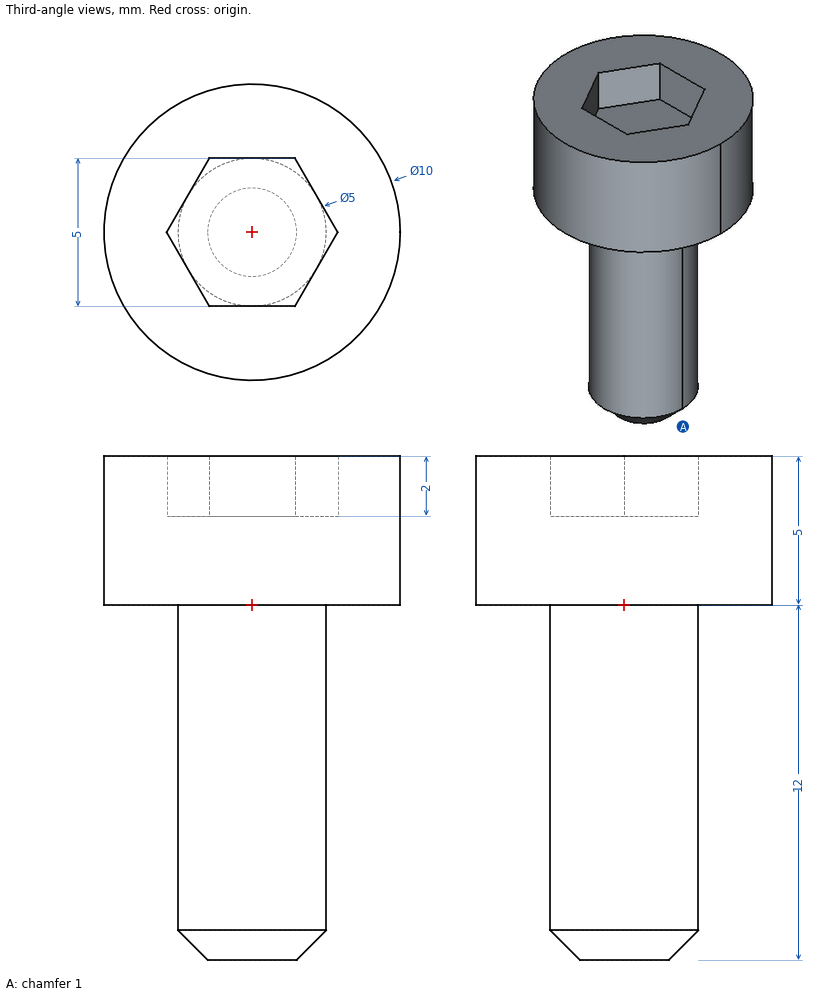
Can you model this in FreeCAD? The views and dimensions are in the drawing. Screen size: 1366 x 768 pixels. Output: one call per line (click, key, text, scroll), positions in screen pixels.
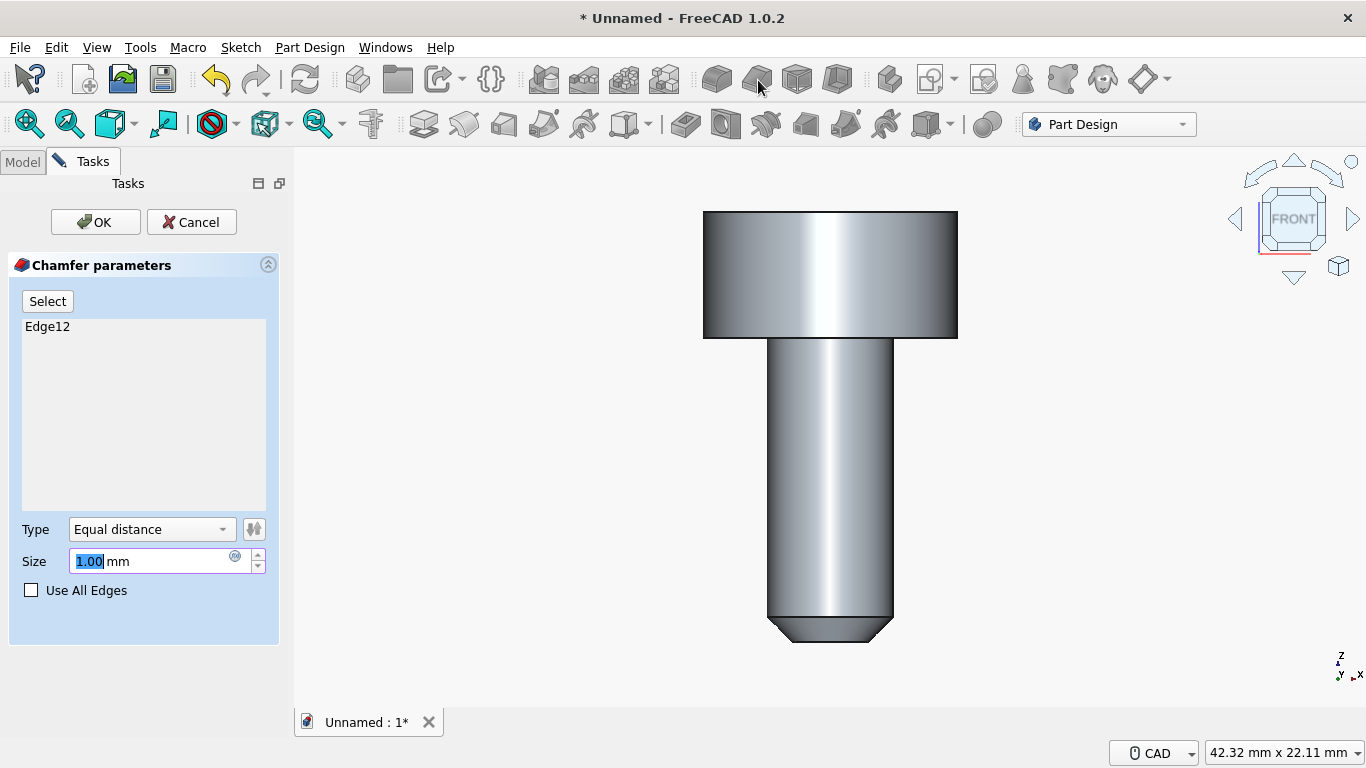
text(1)
key(Tab)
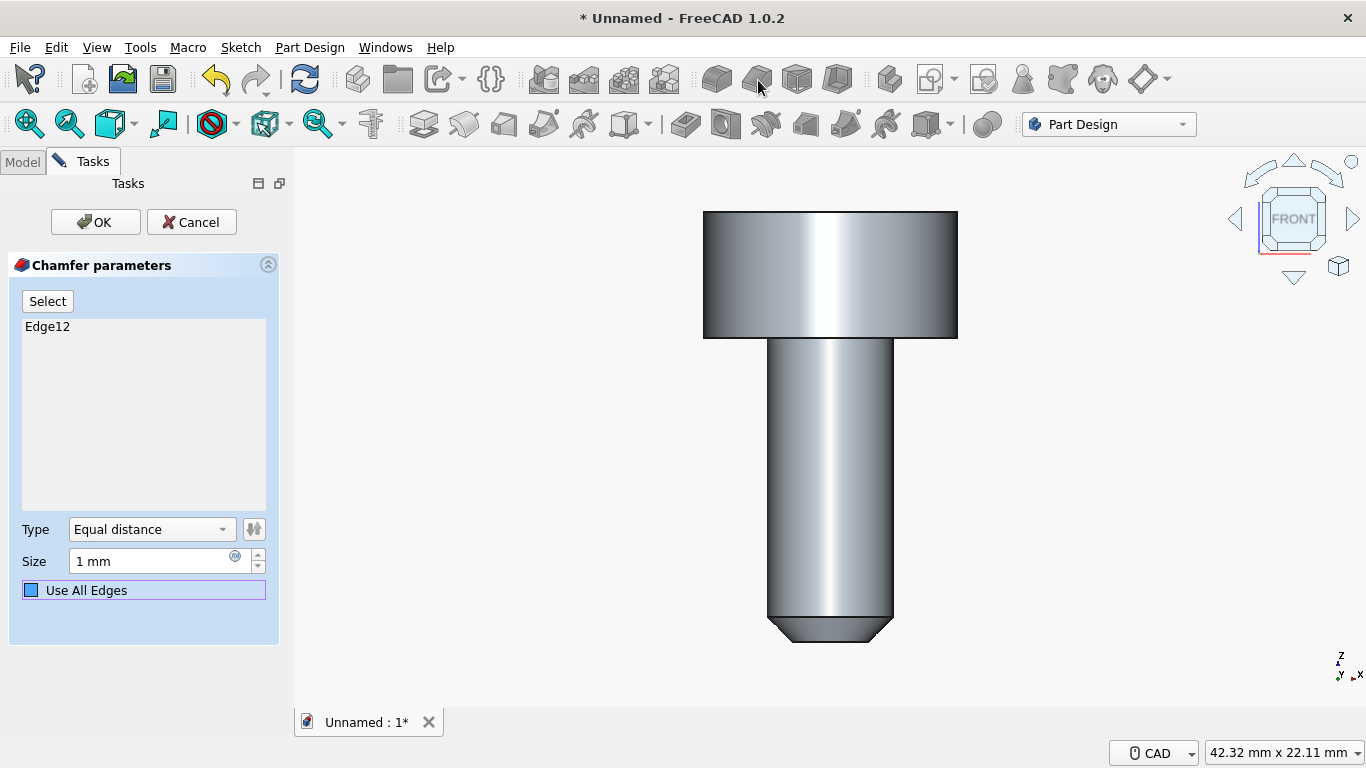
click(96, 222)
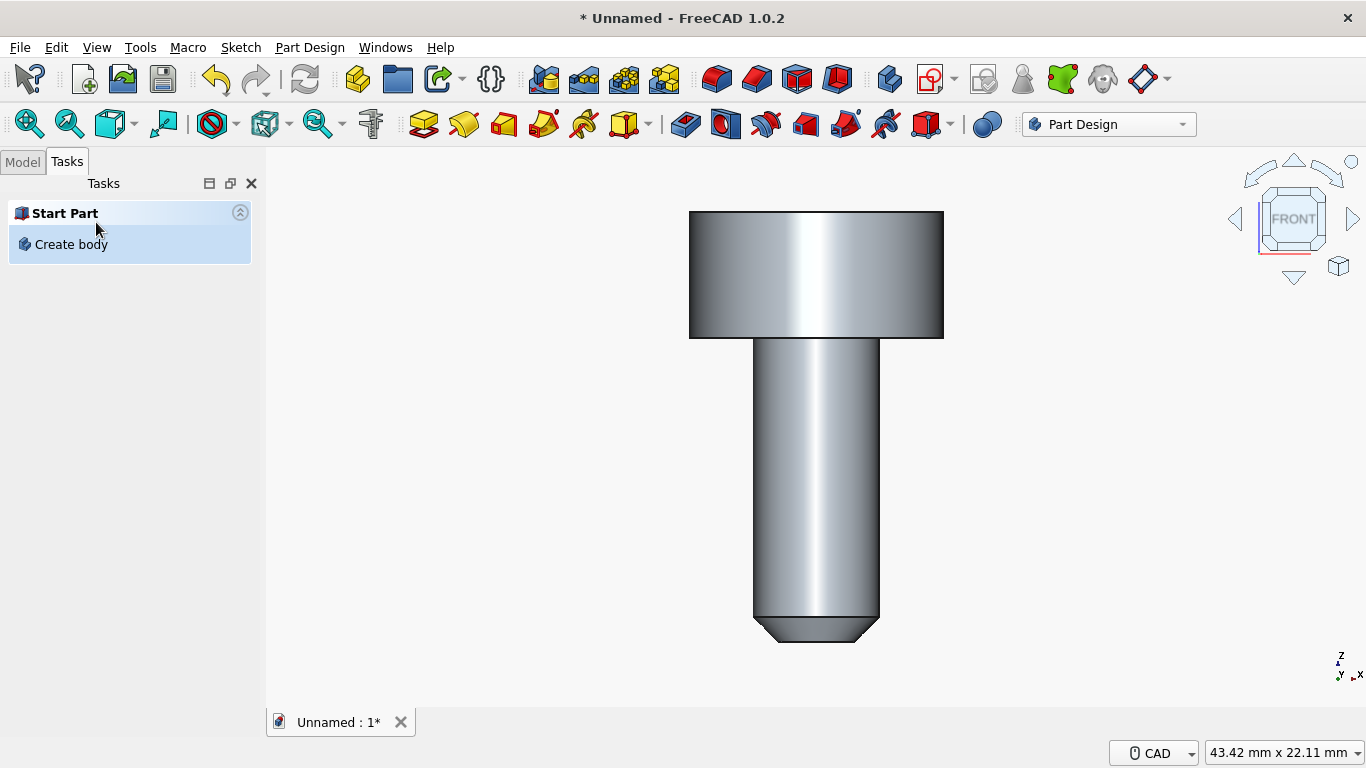
key(0)